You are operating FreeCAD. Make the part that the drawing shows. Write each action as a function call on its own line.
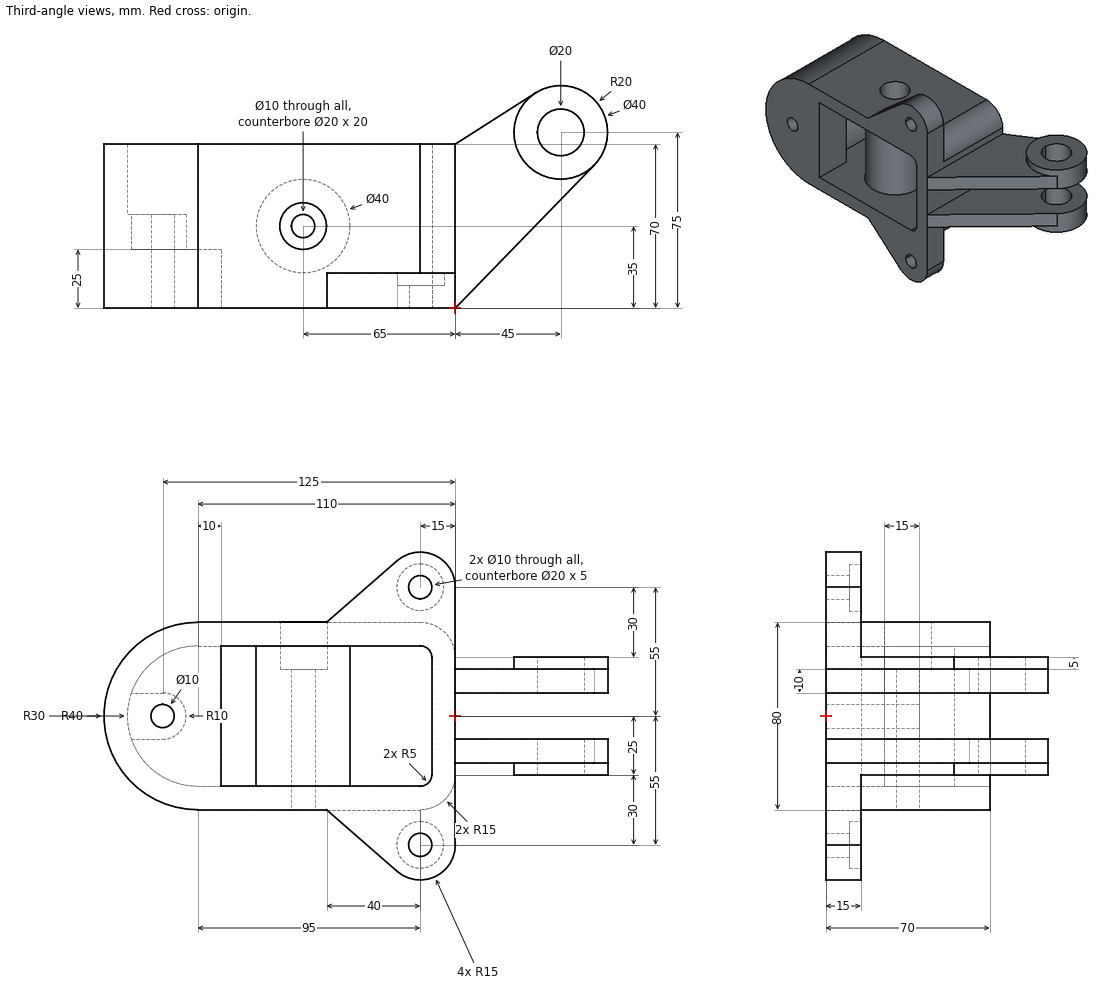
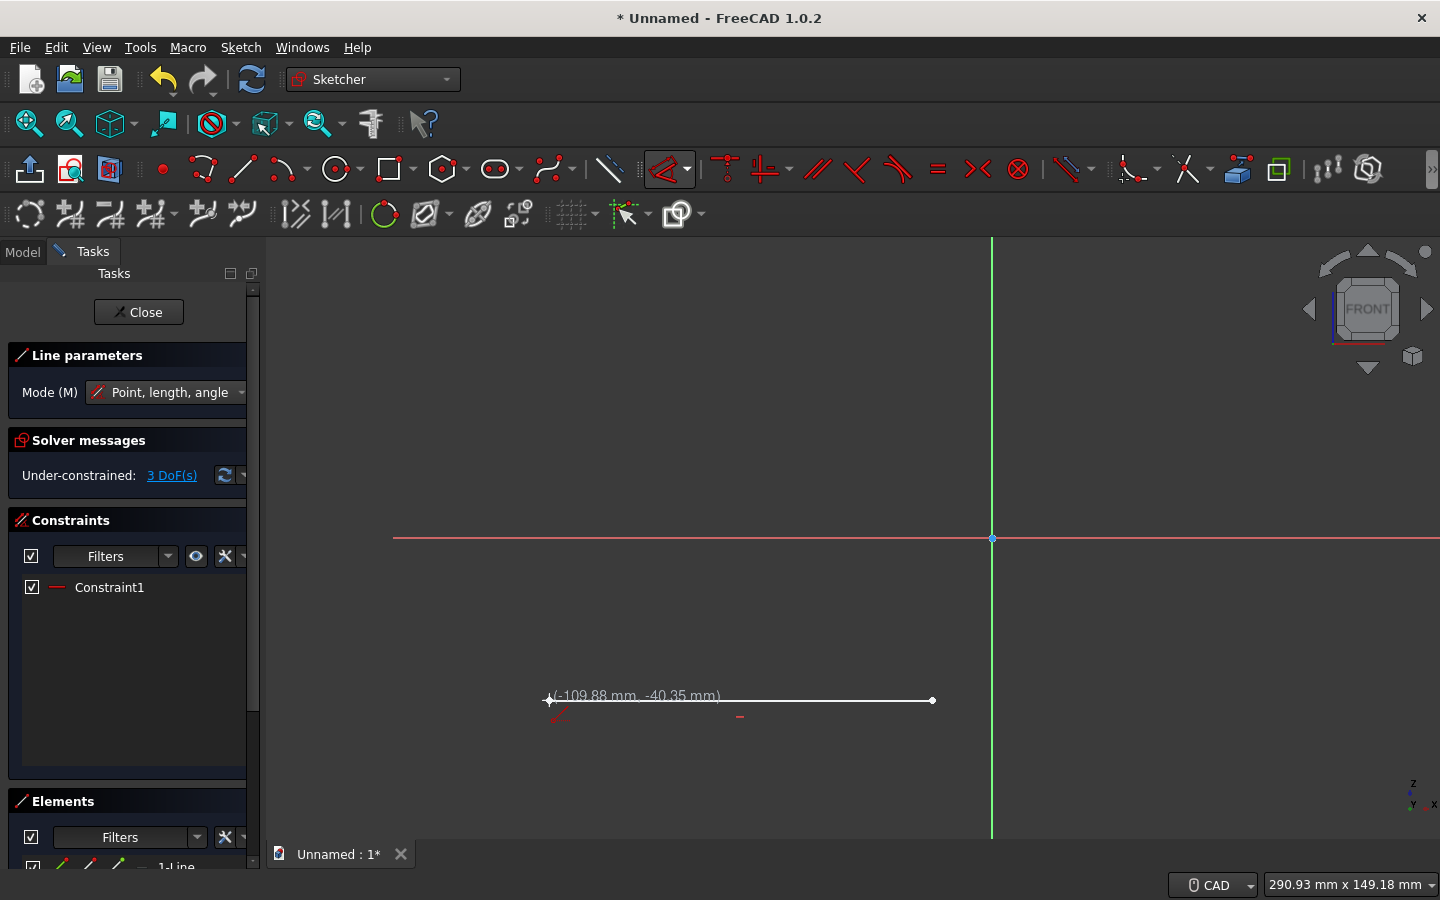
click(549, 377)
click(932, 377)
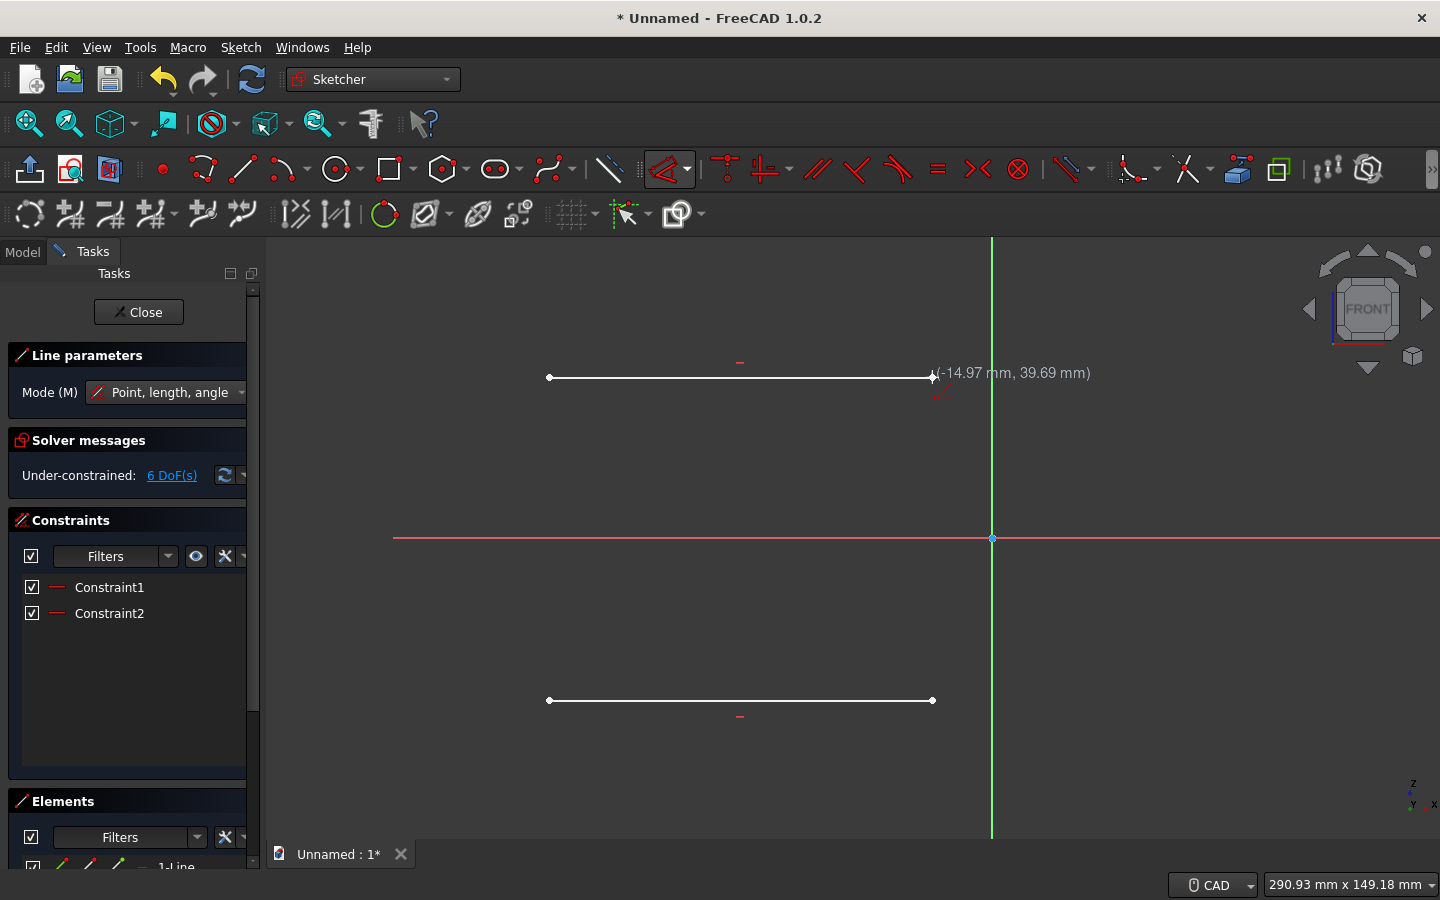
click(992, 437)
click(983, 639)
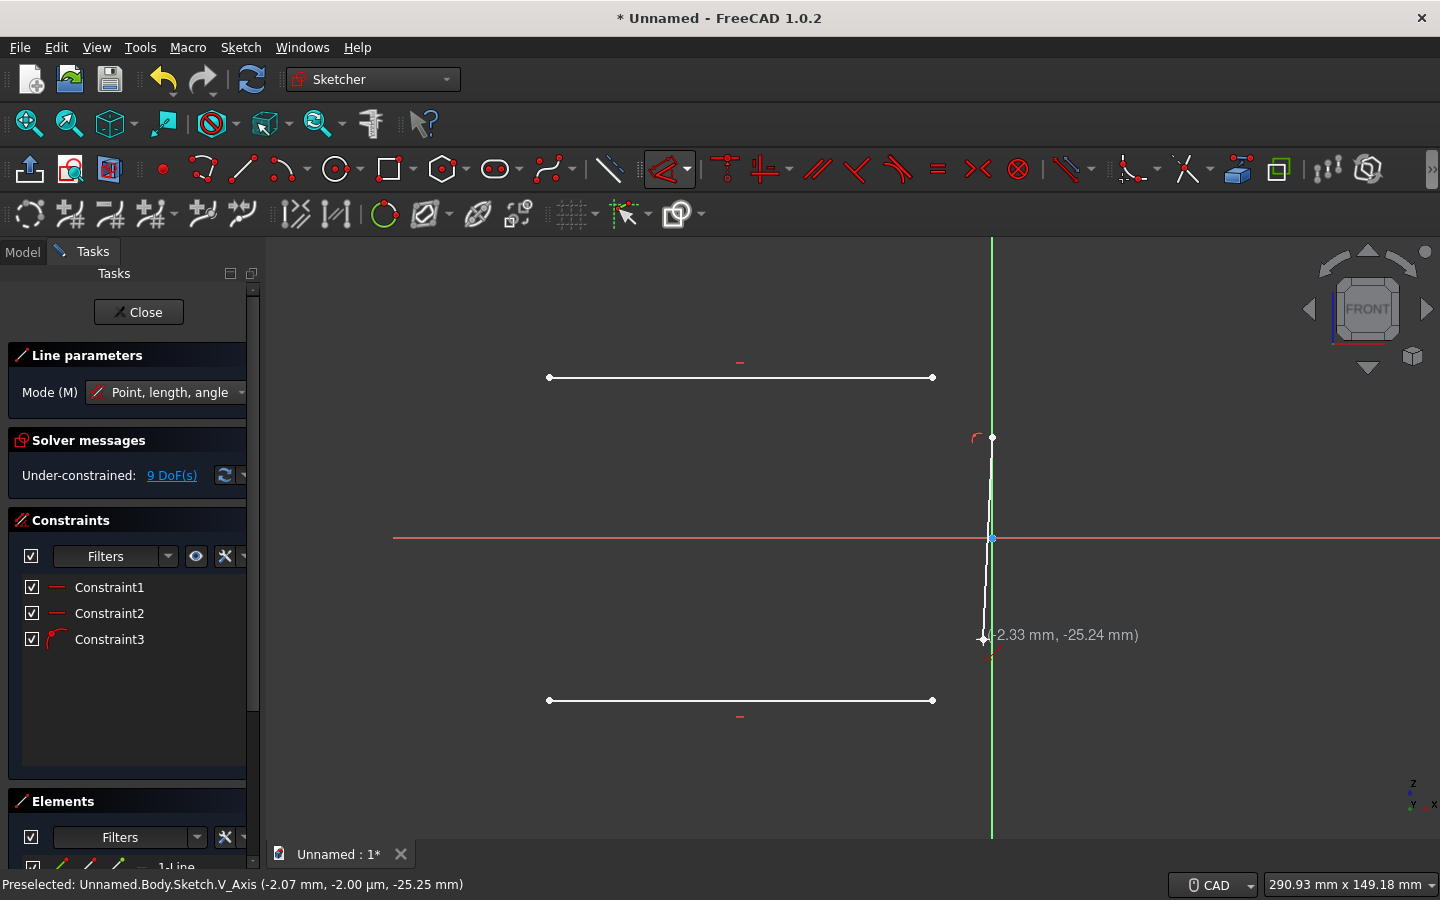
key(g)
key(3)
key(a)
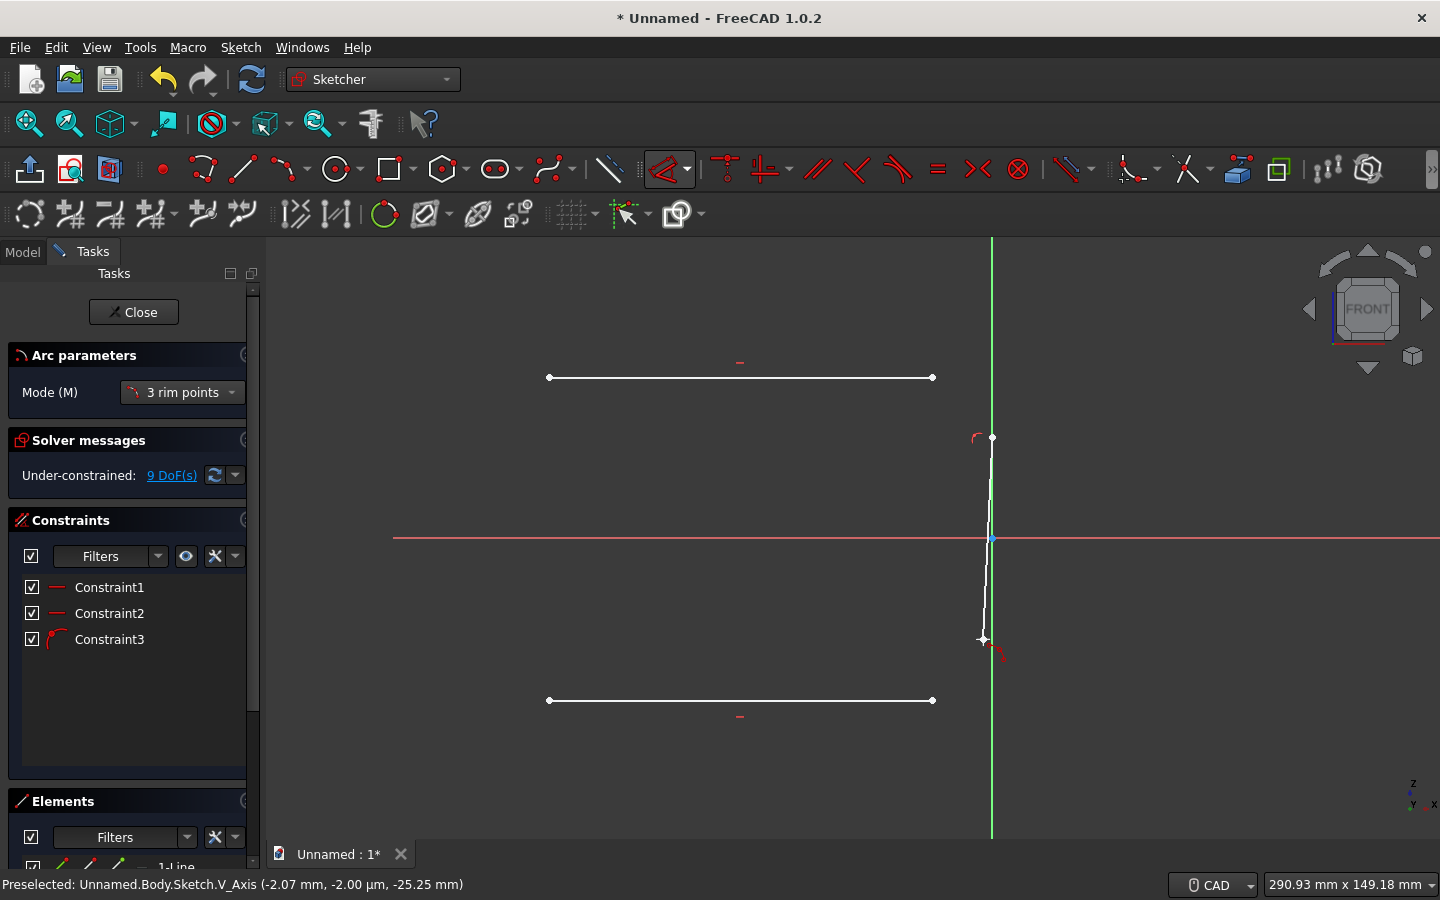
click(549, 701)
click(549, 378)
click(395, 488)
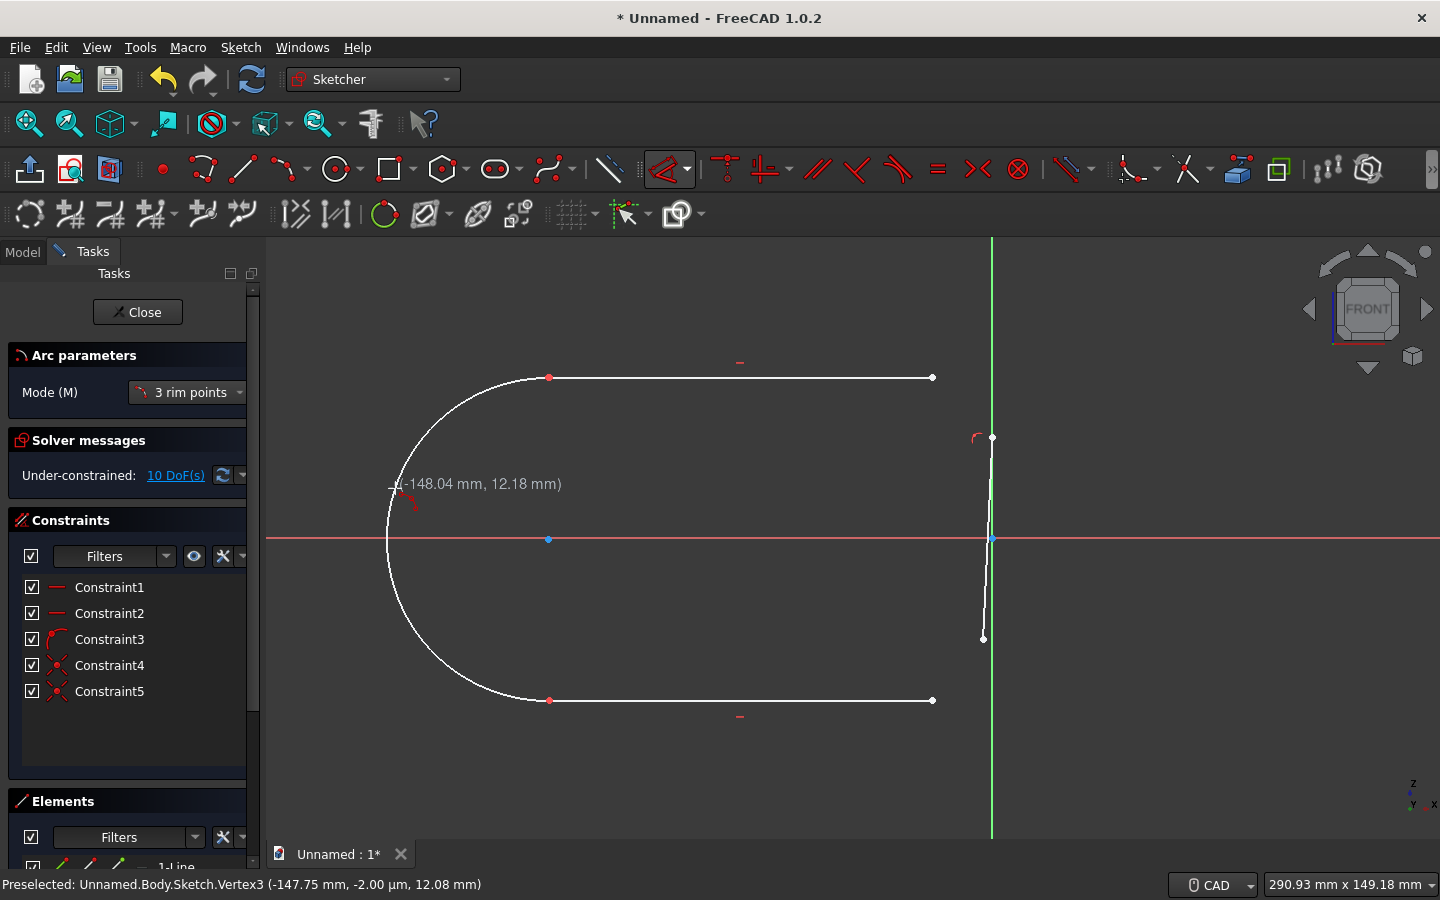
click(932, 378)
click(992, 438)
click(975, 394)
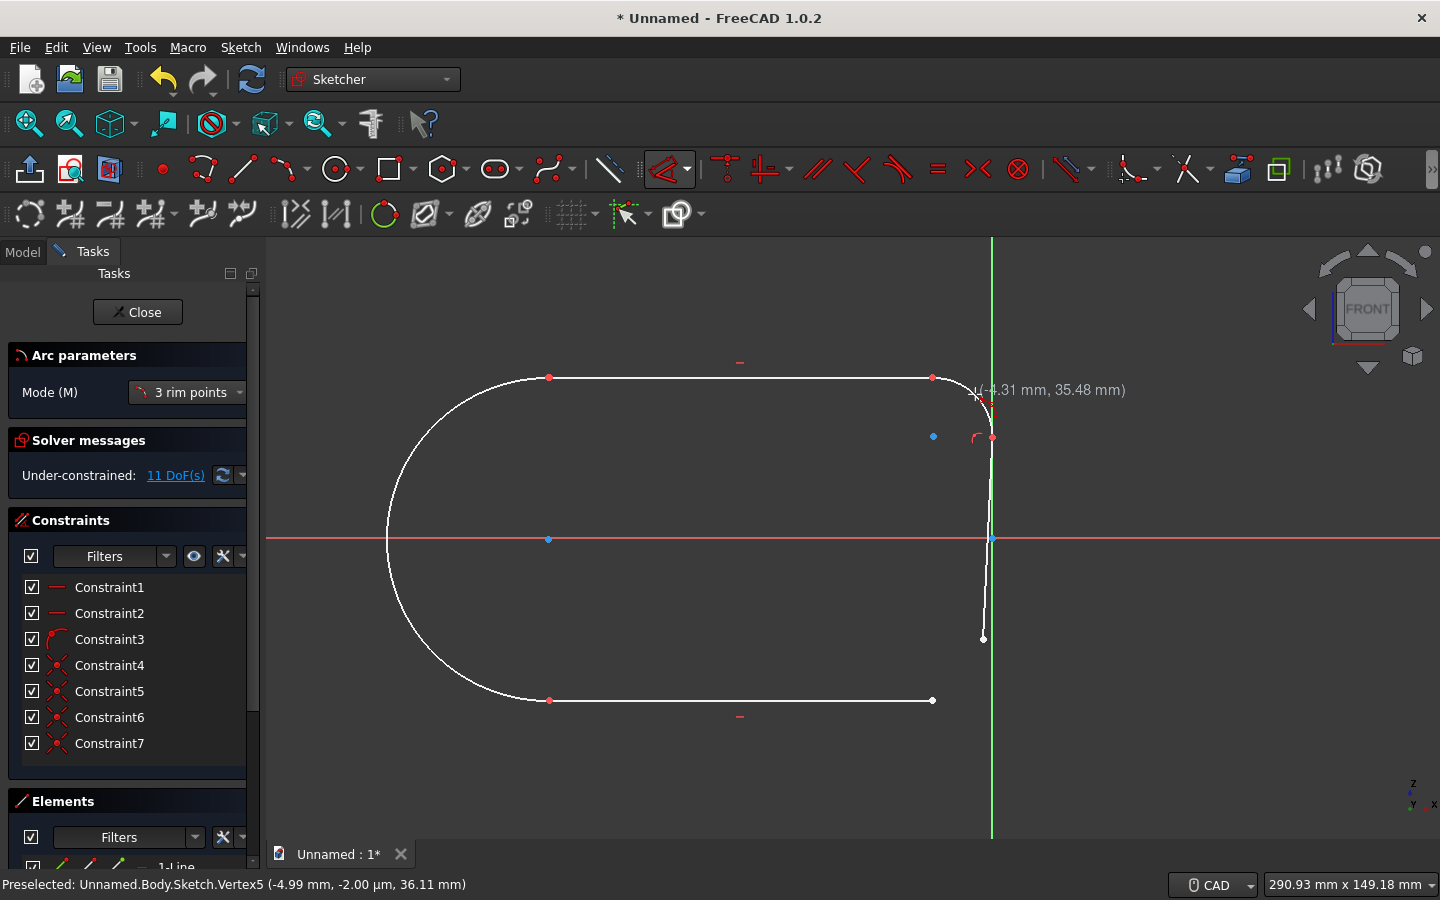
click(983, 640)
click(932, 701)
click(975, 682)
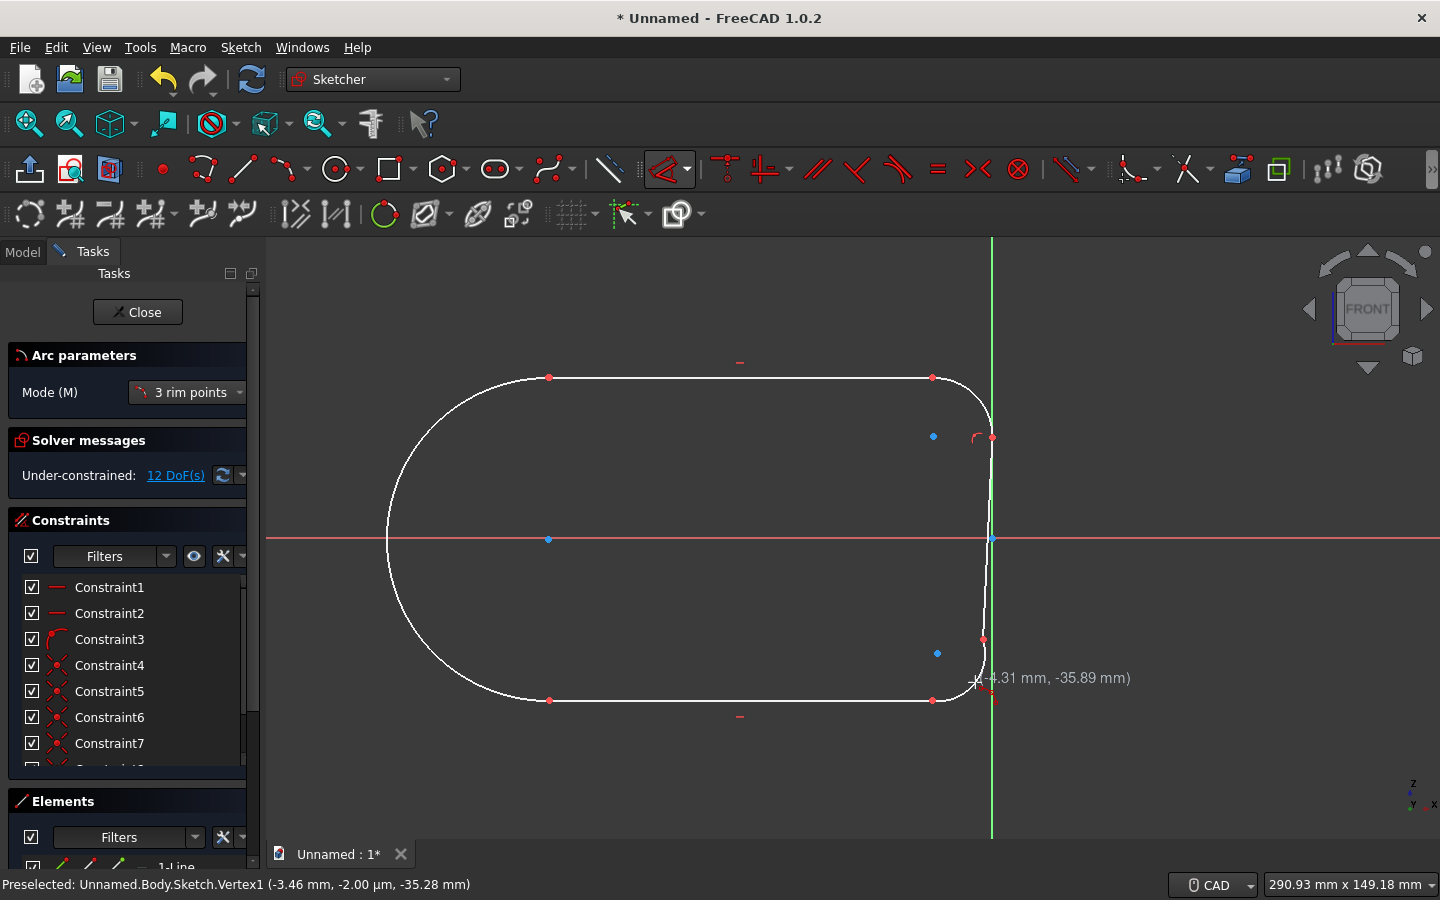
key(g)
key(l)